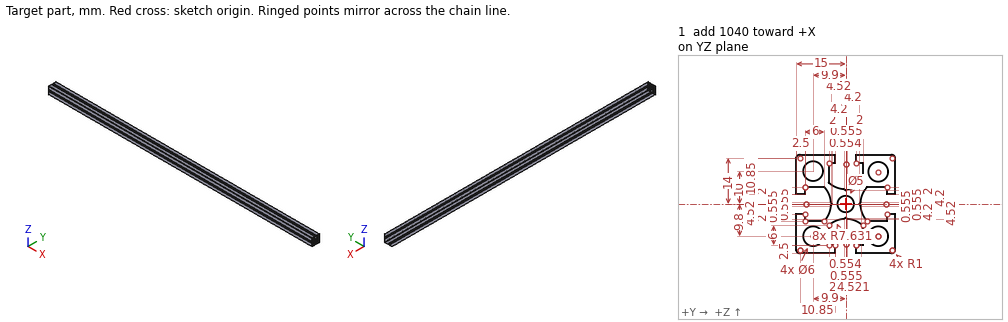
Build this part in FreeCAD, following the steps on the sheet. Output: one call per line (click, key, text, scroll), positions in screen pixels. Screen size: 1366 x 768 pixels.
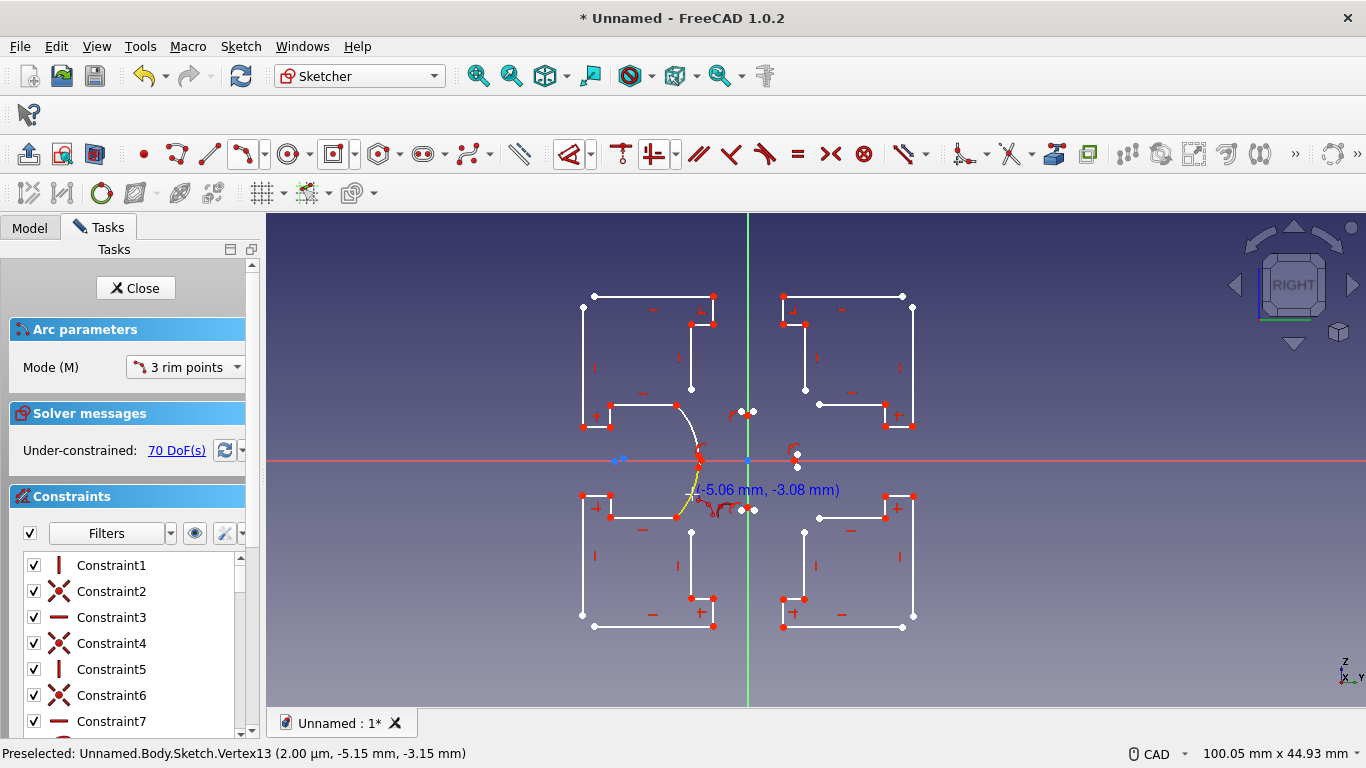
click(583, 616)
click(594, 627)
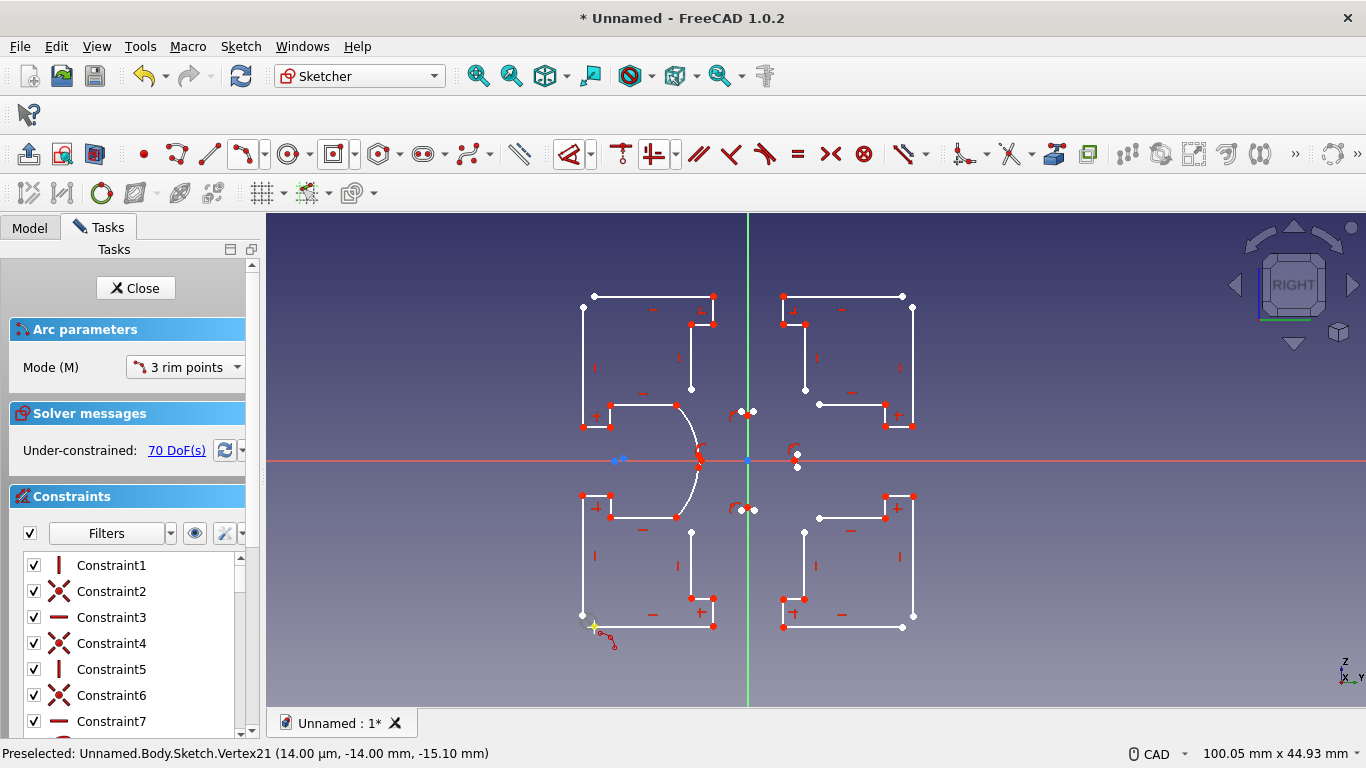
scroll(586, 622, up, 8)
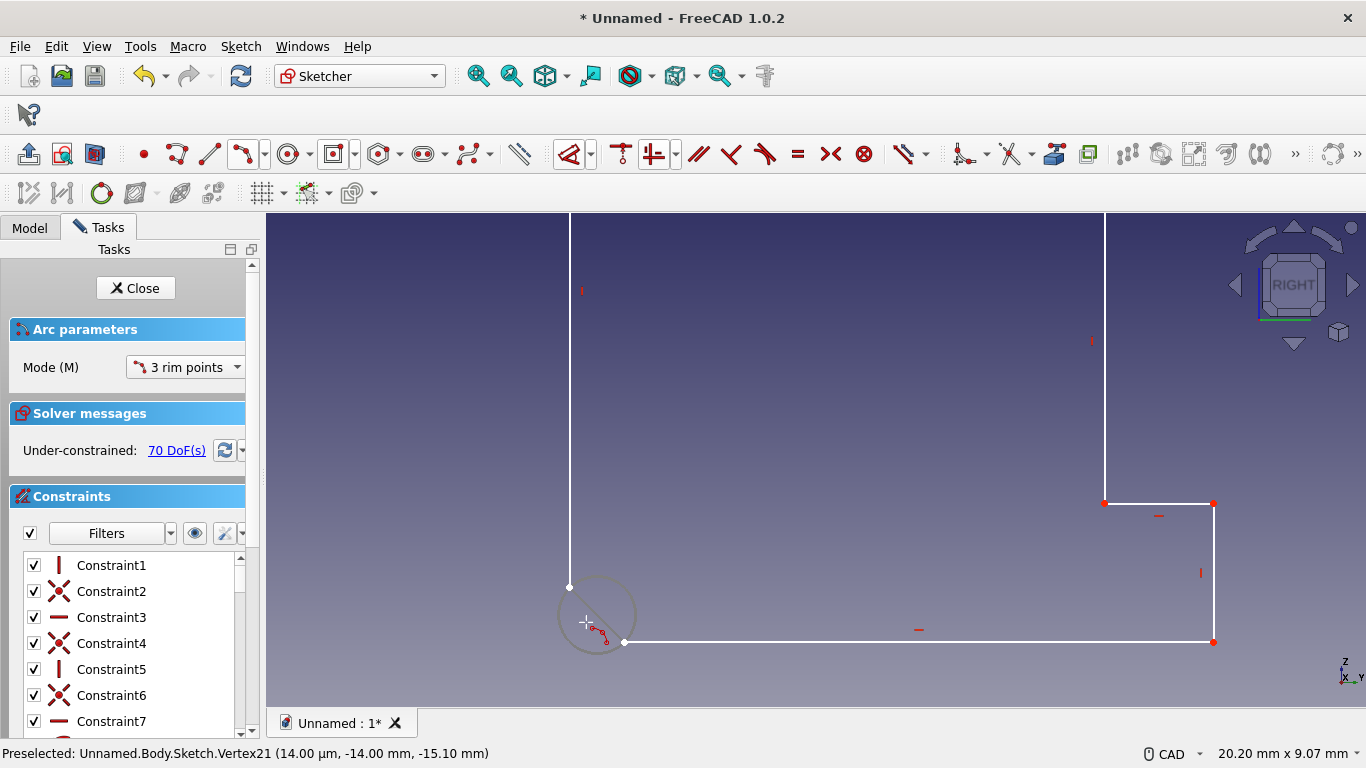
click(586, 621)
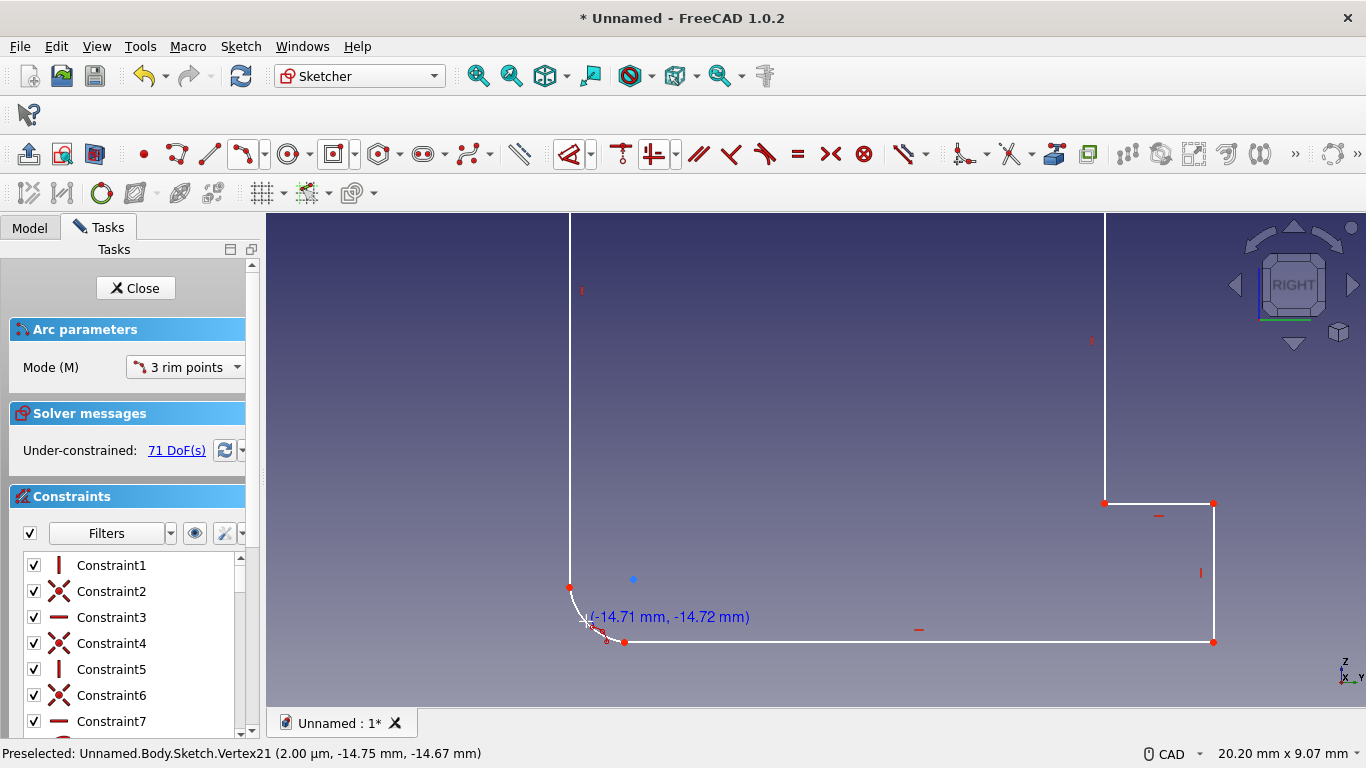
scroll(586, 622, down, 8)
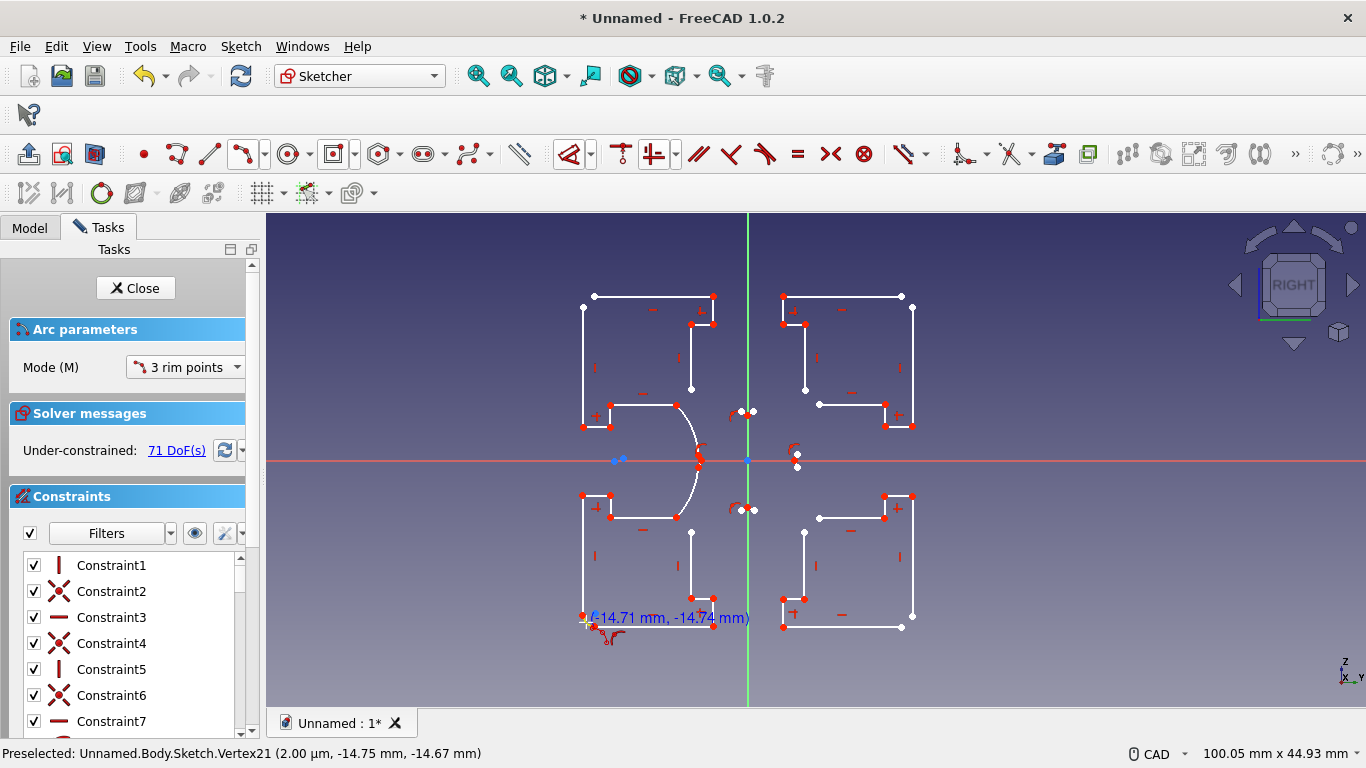
click(691, 533)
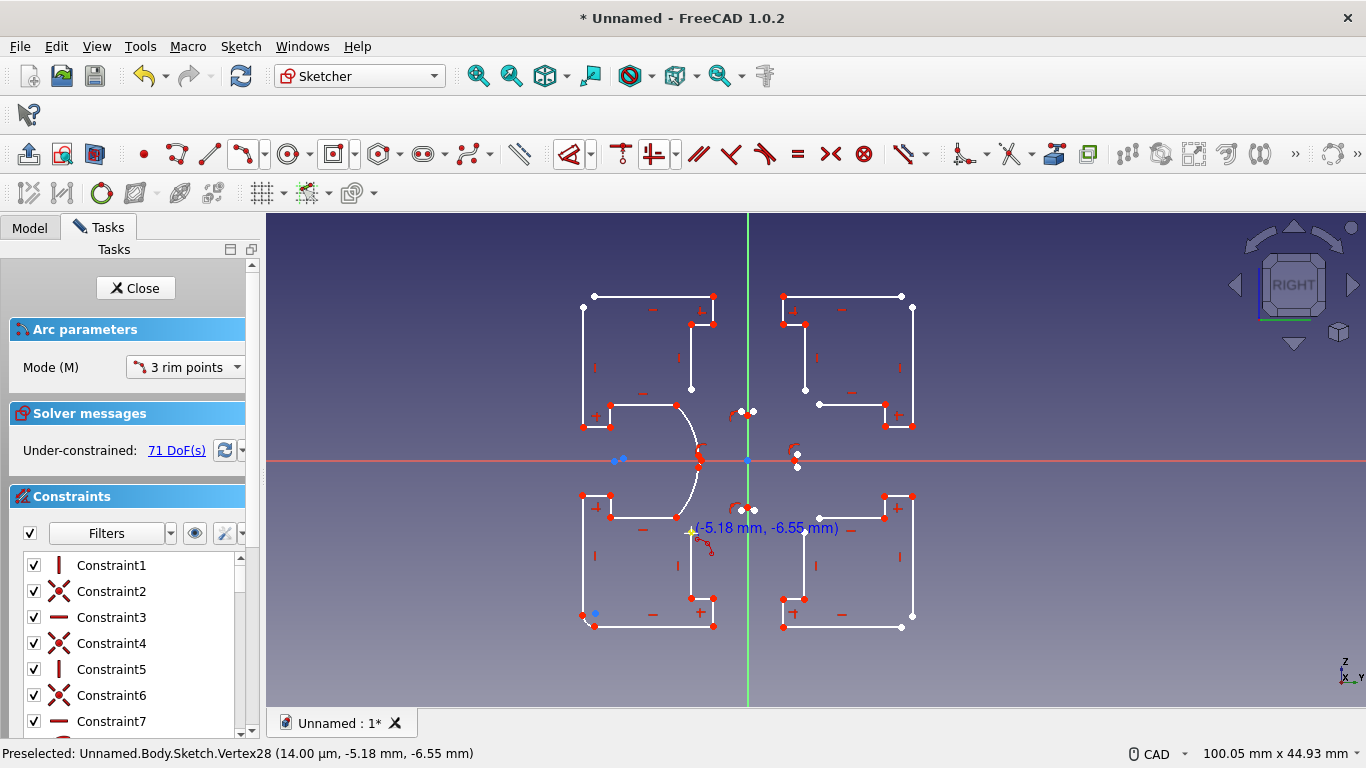
scroll(742, 510, up, 8)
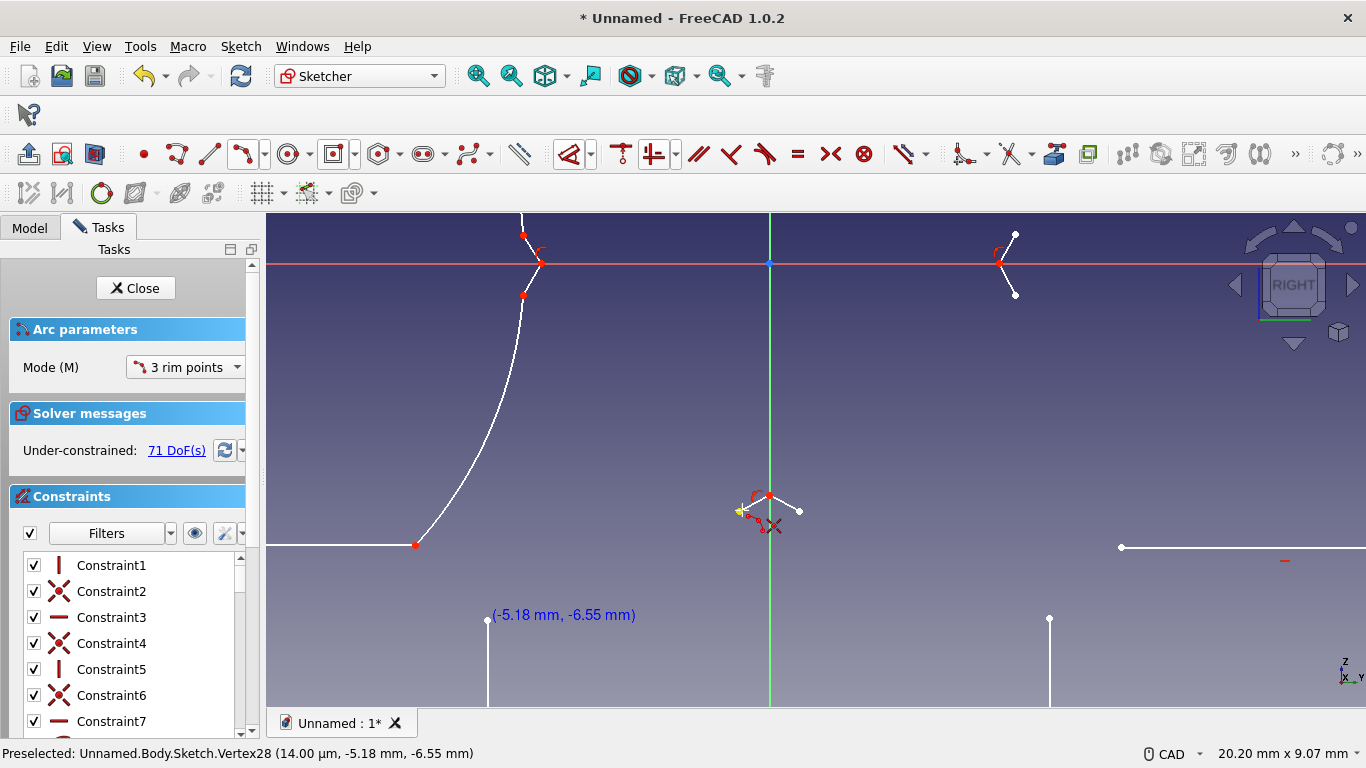
click(740, 511)
click(605, 543)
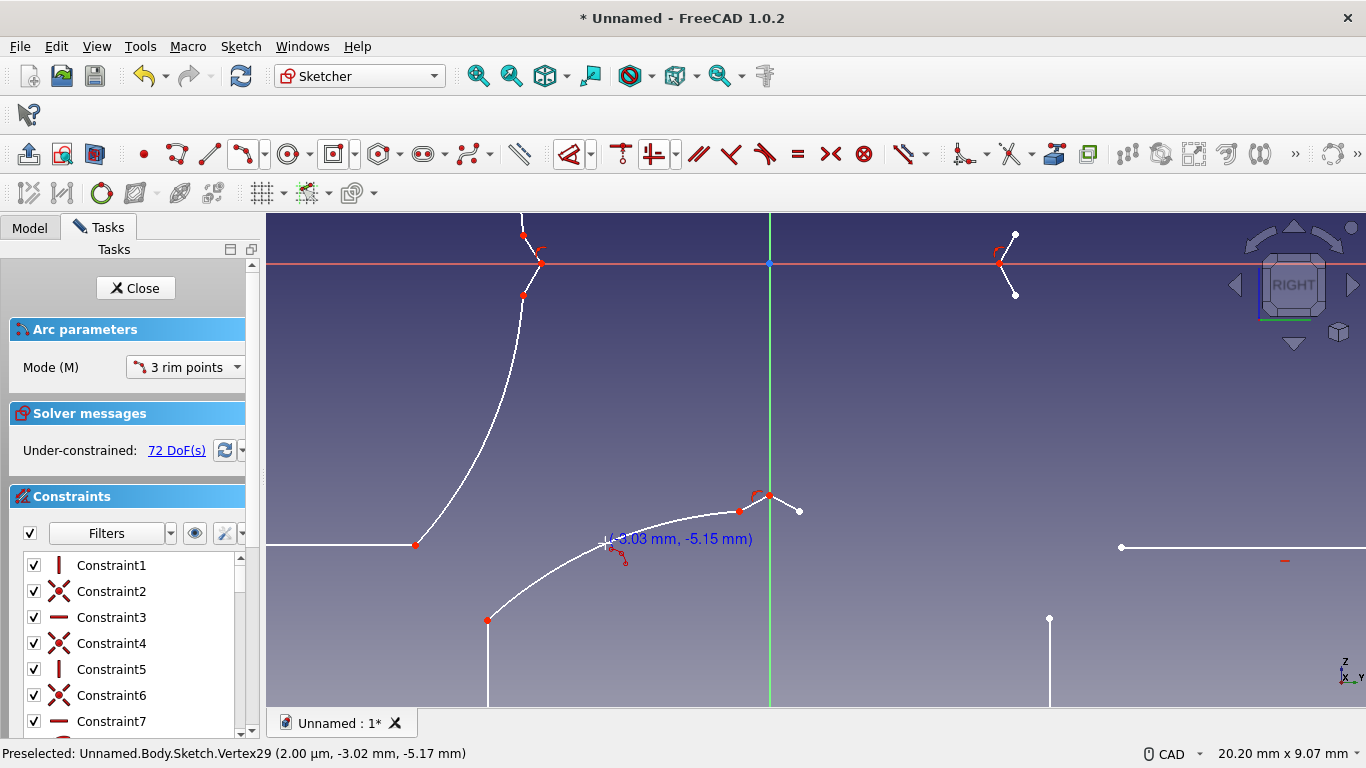
click(800, 511)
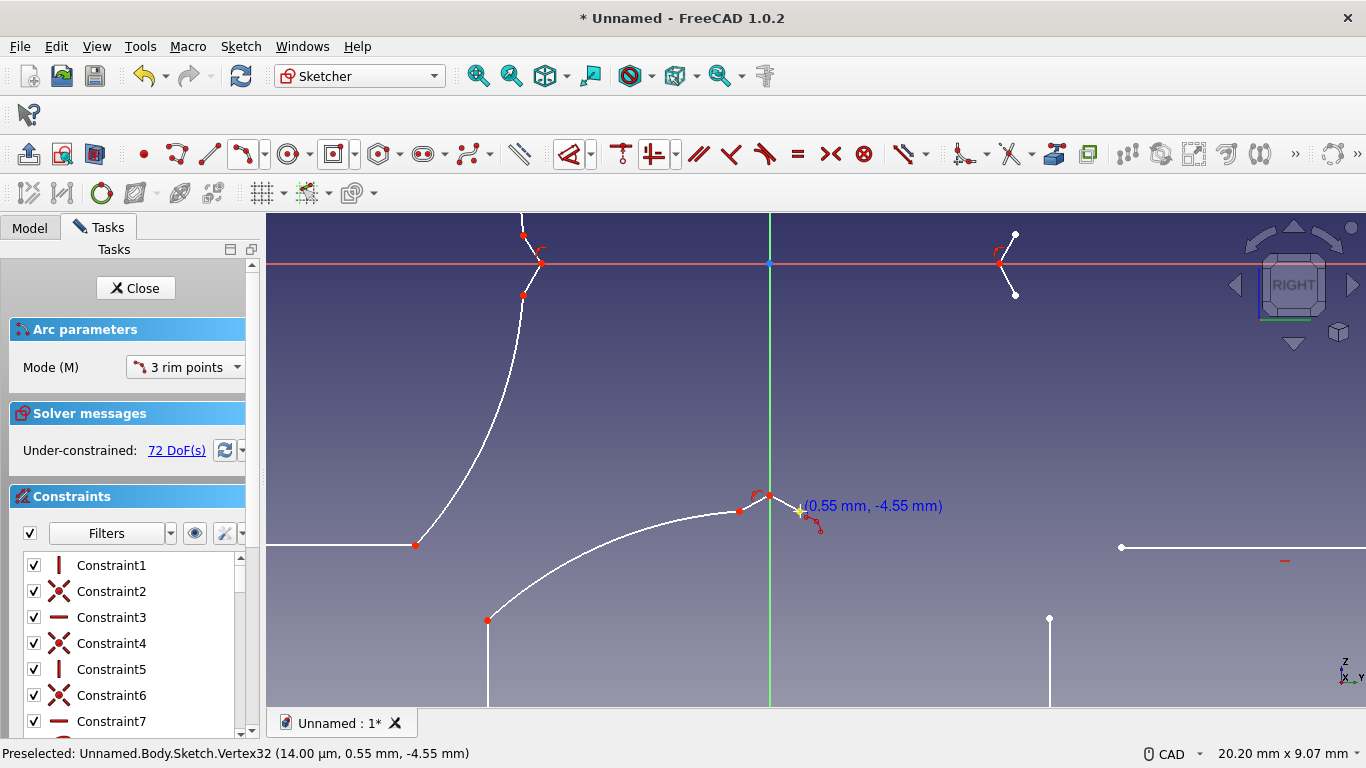
scroll(742, 510, down, 8)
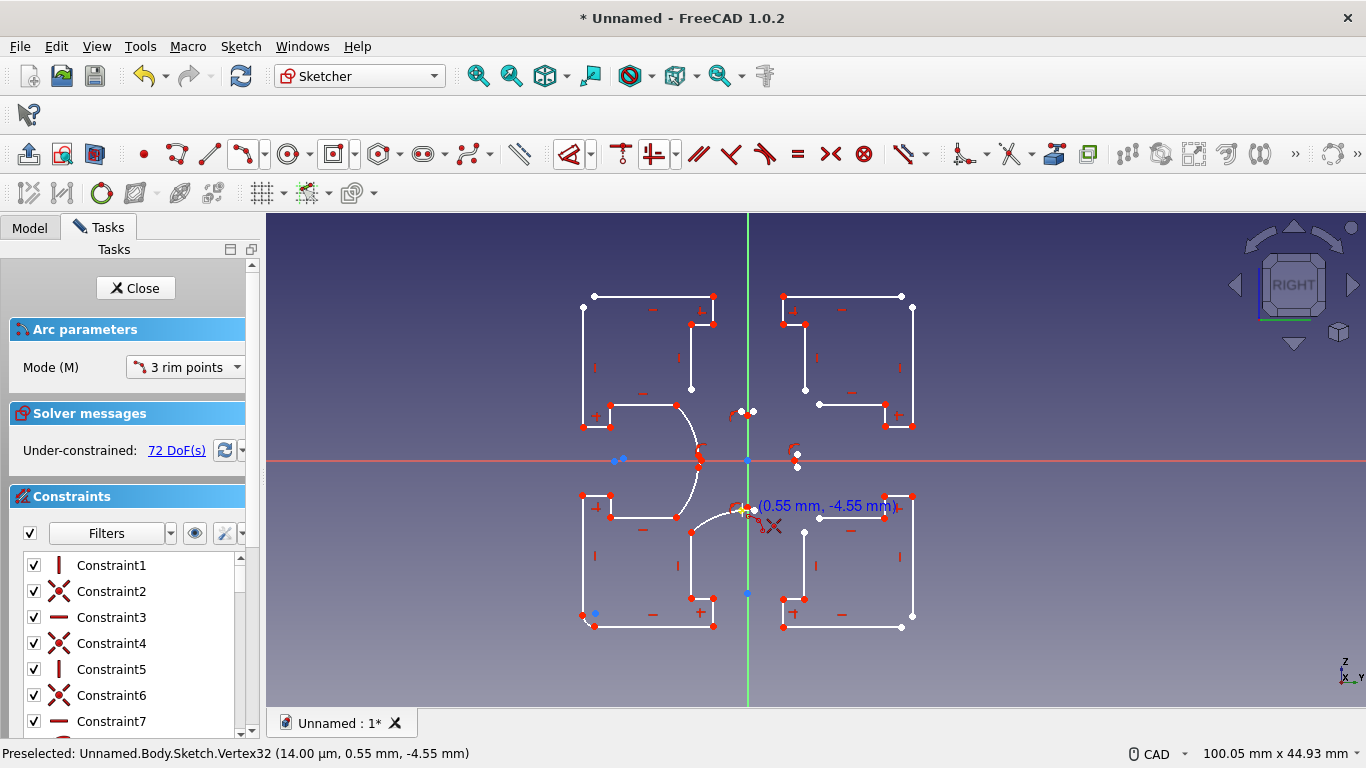
click(804, 532)